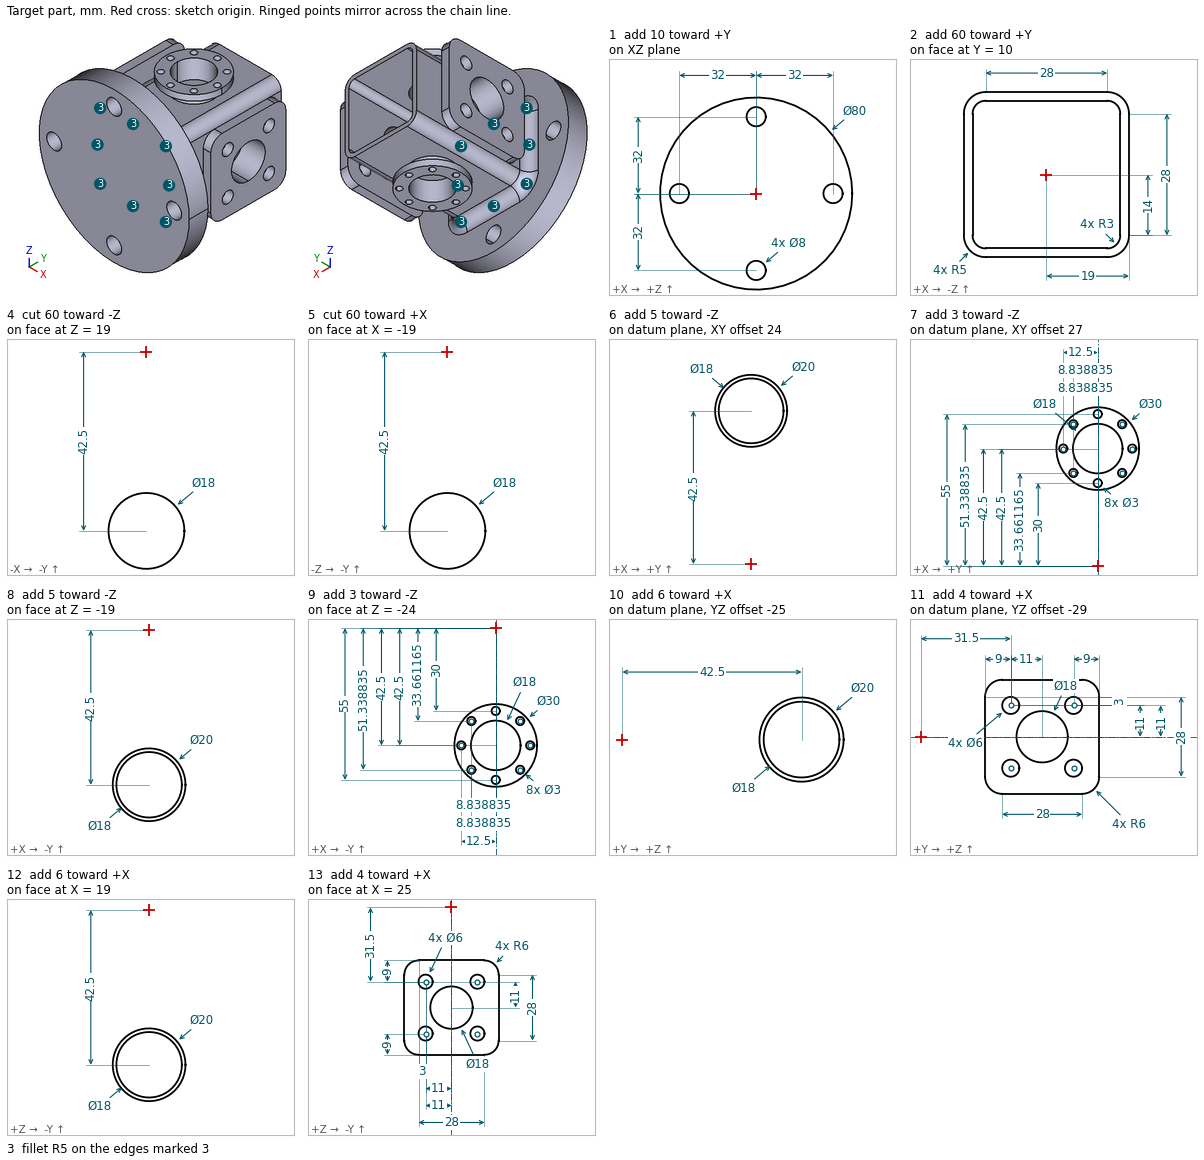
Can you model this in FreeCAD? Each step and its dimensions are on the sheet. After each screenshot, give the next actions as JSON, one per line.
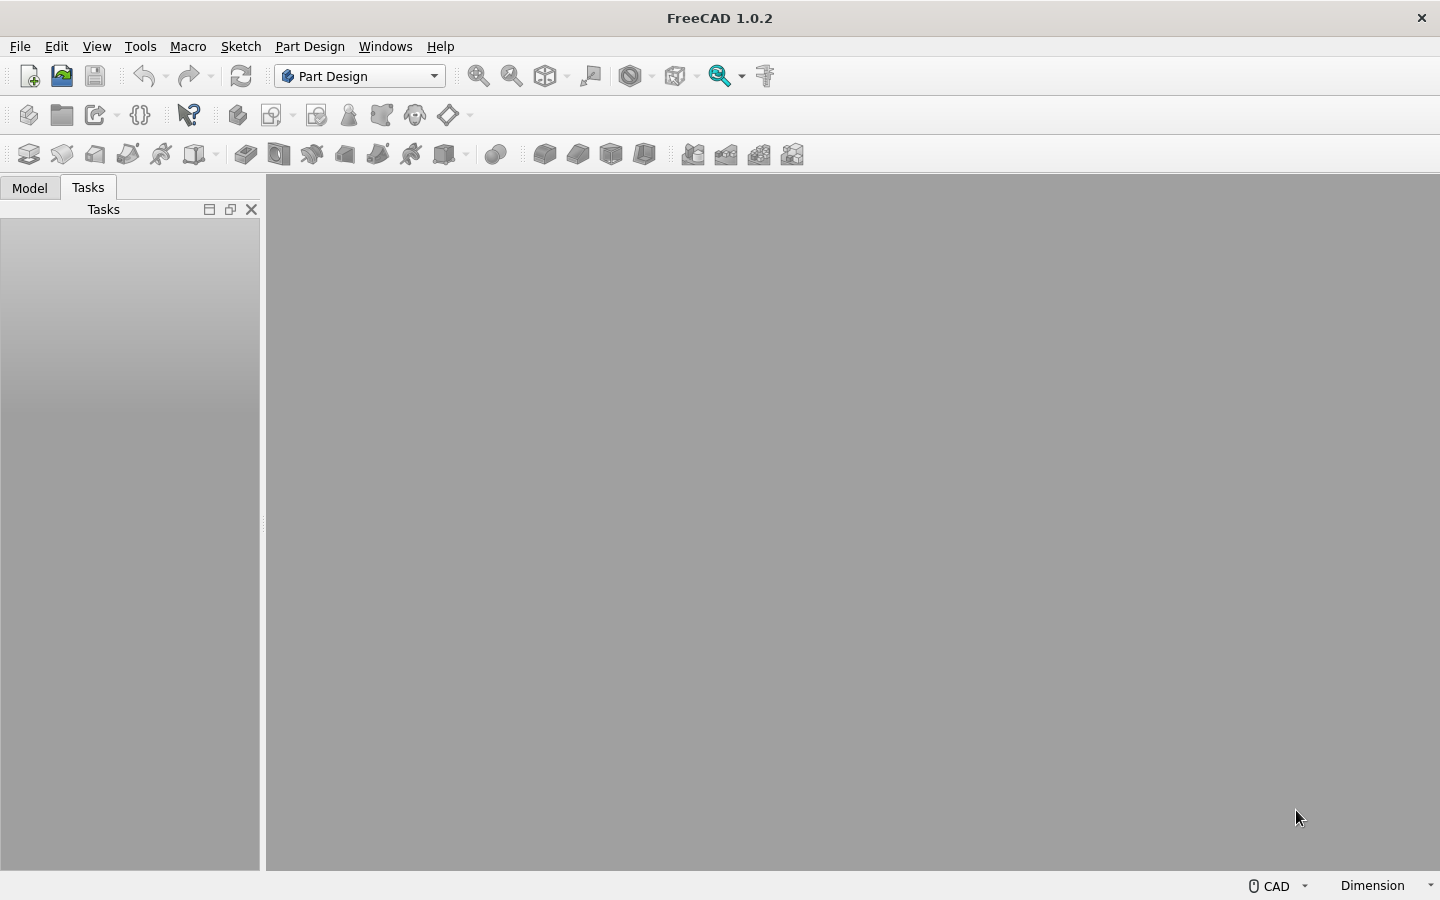
{"action": "key", "text": "ctrl+n"}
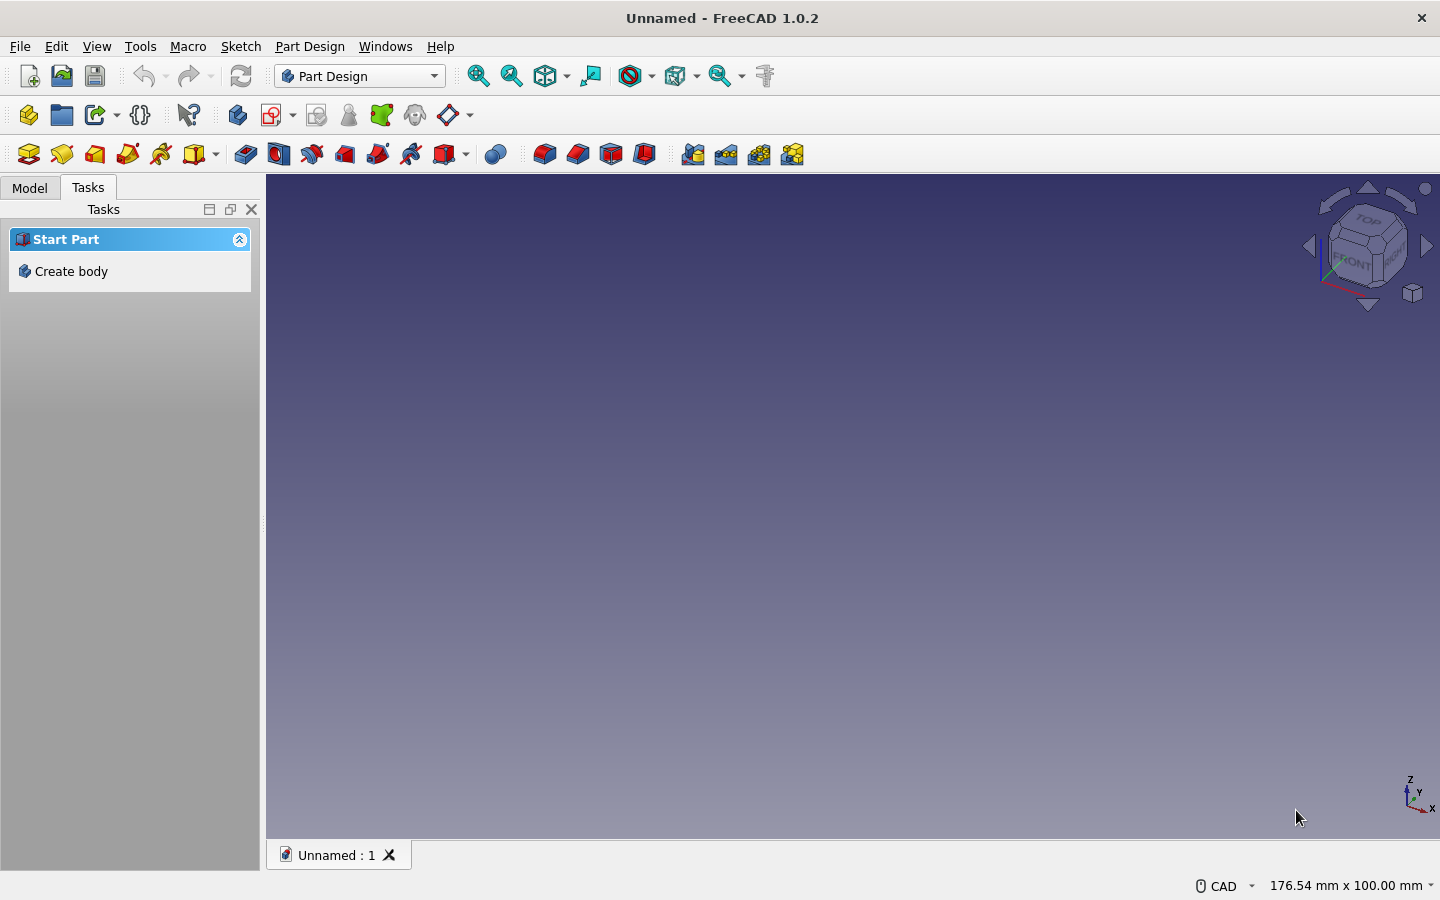
{"action": "left_click", "coordinate": [270, 116]}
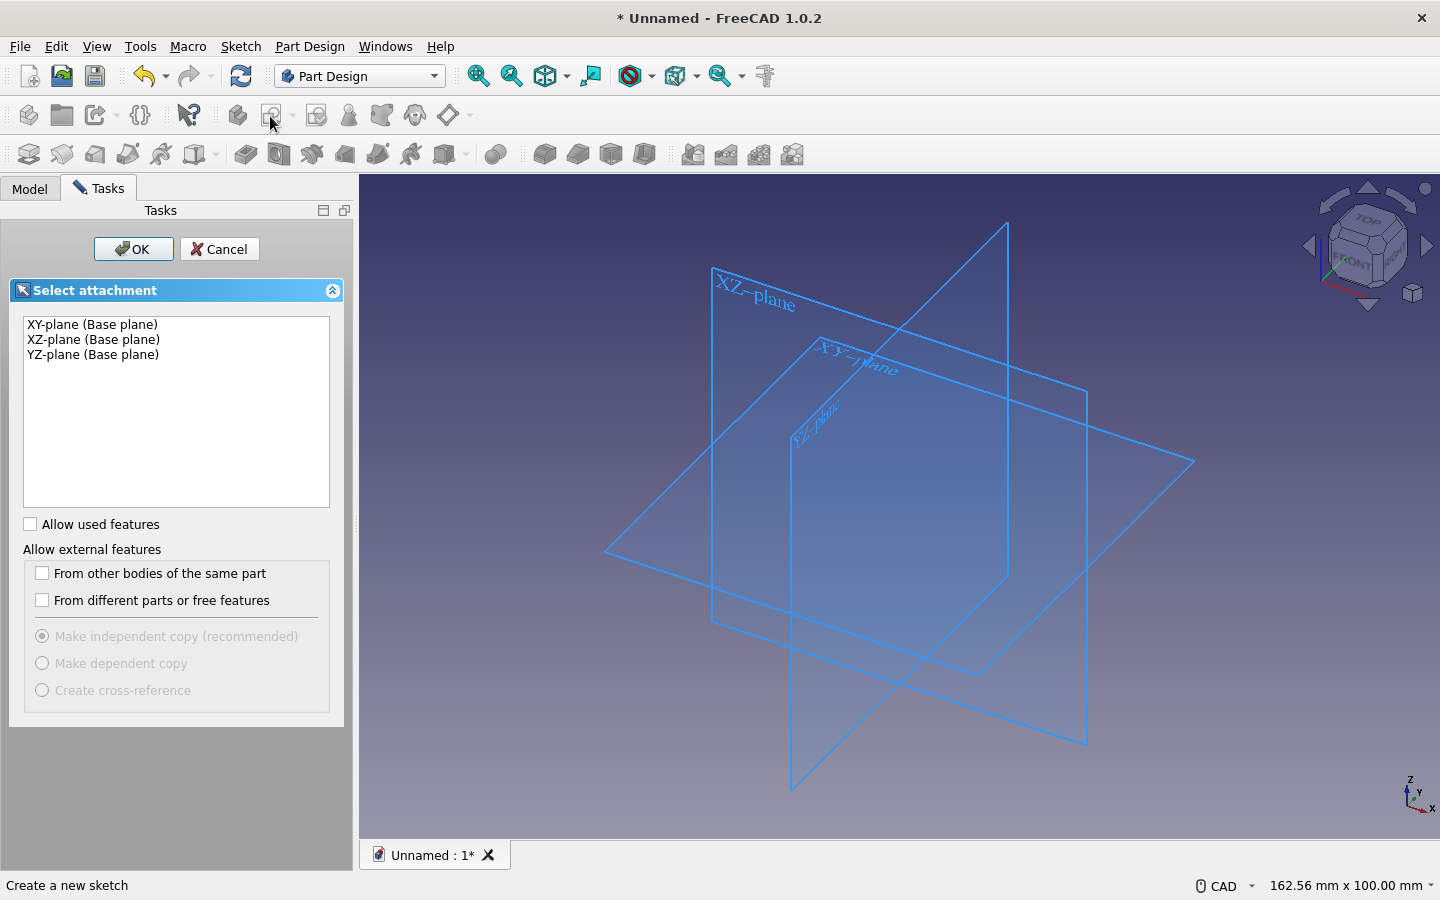
{"action": "left_click", "coordinate": [84, 340]}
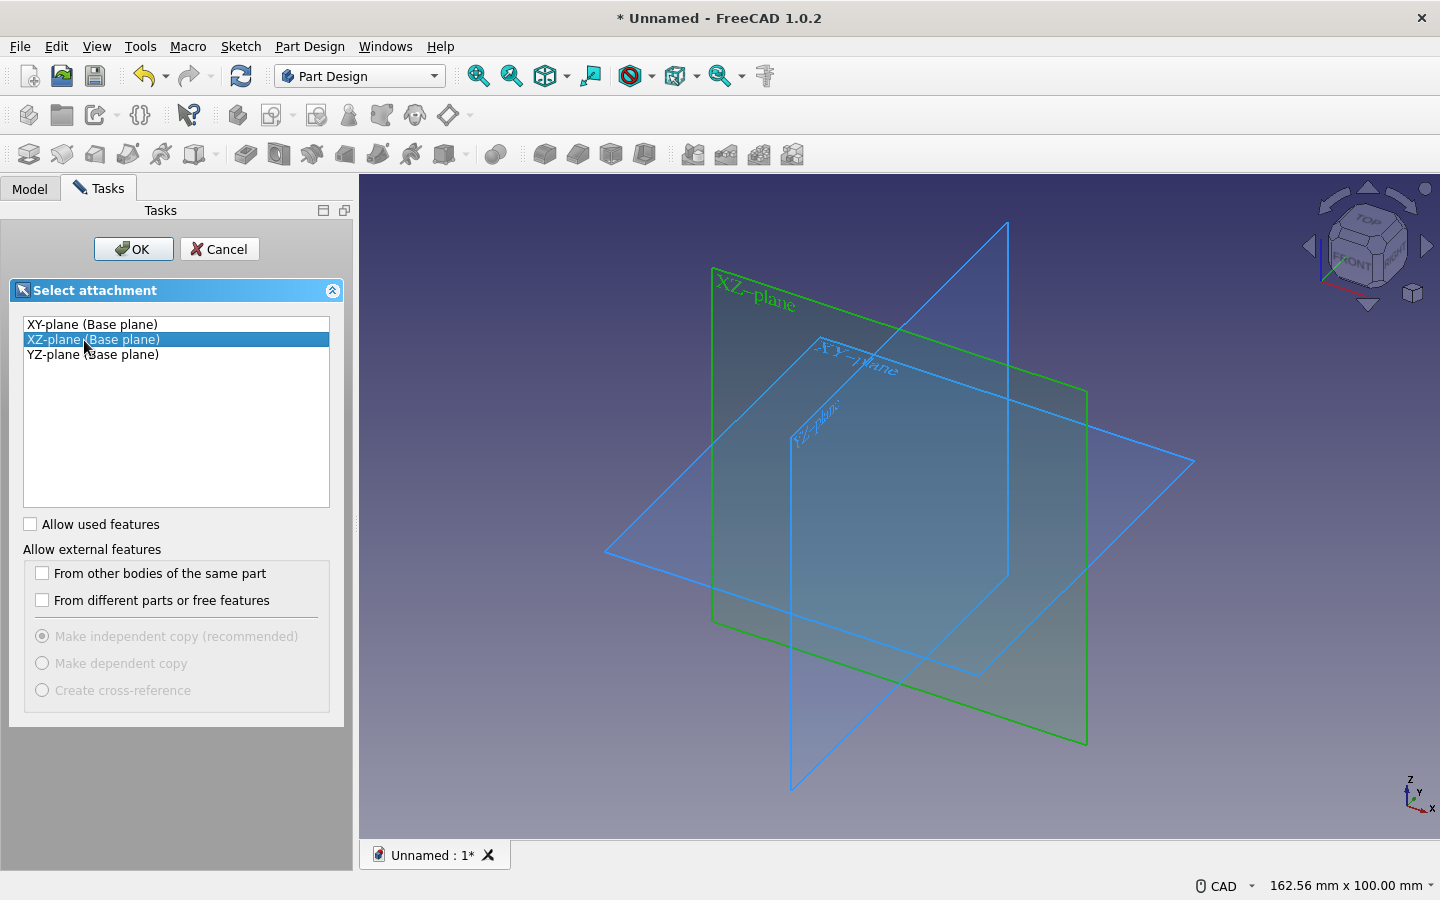
{"action": "left_click", "coordinate": [134, 249]}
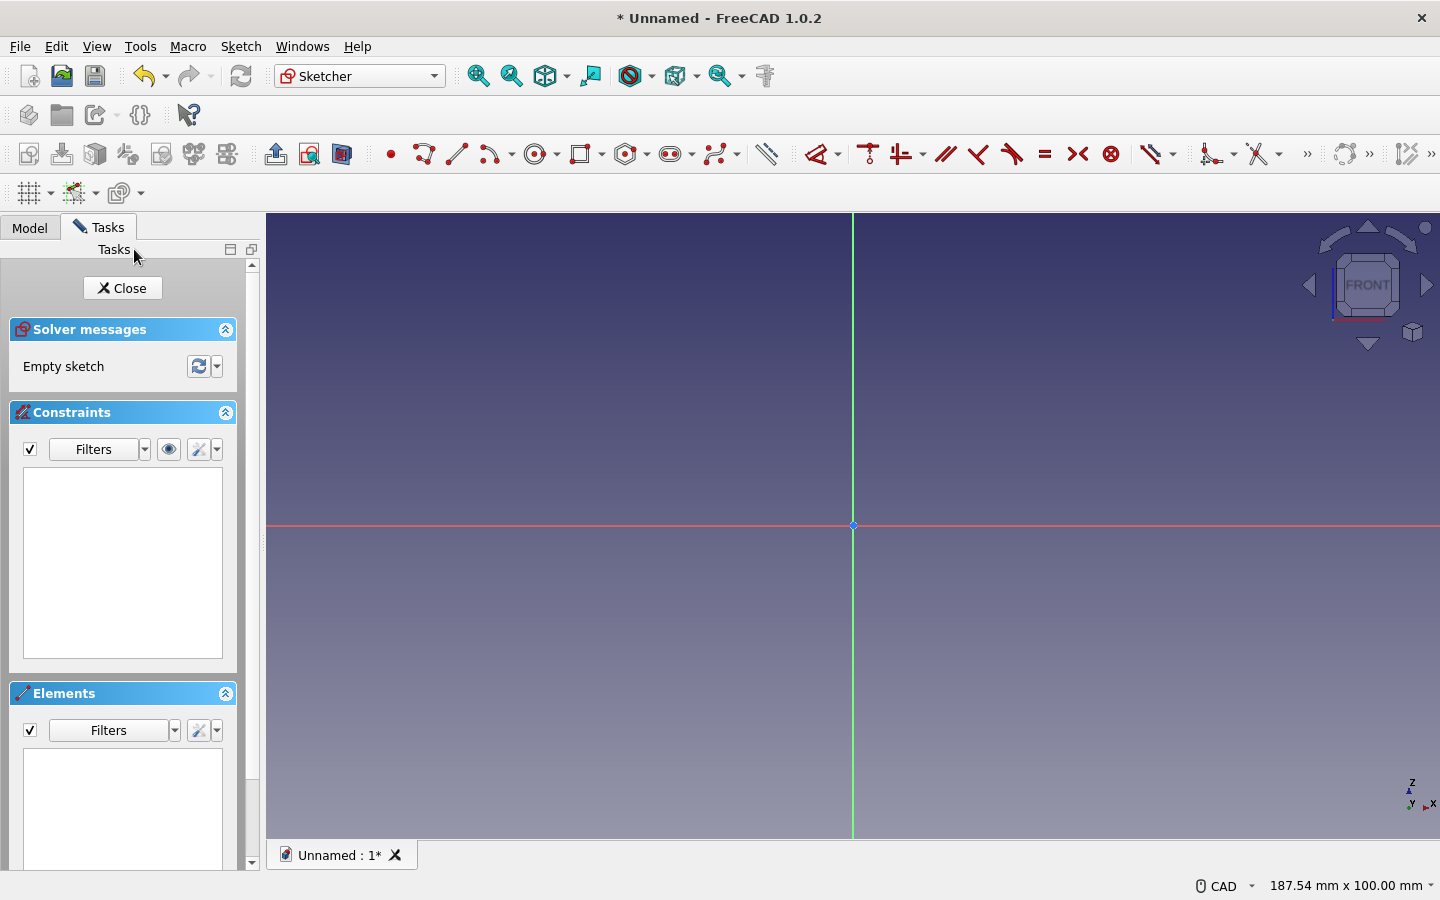
{"action": "left_click", "coordinate": [534, 154]}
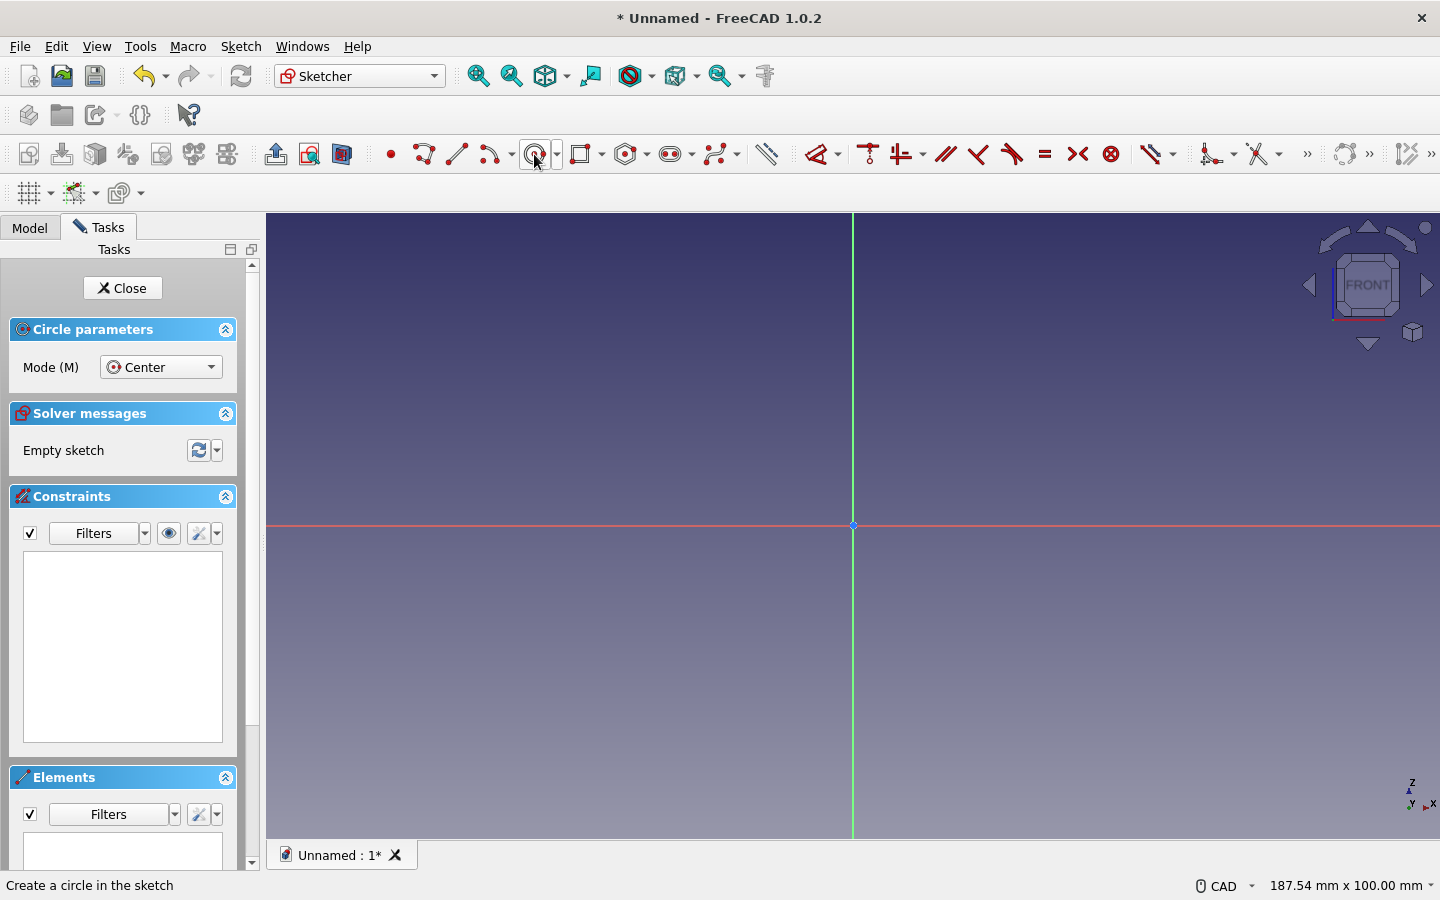
{"action": "left_click", "coordinate": [853, 526]}
{"action": "mouse_move", "coordinate": [1030, 349]}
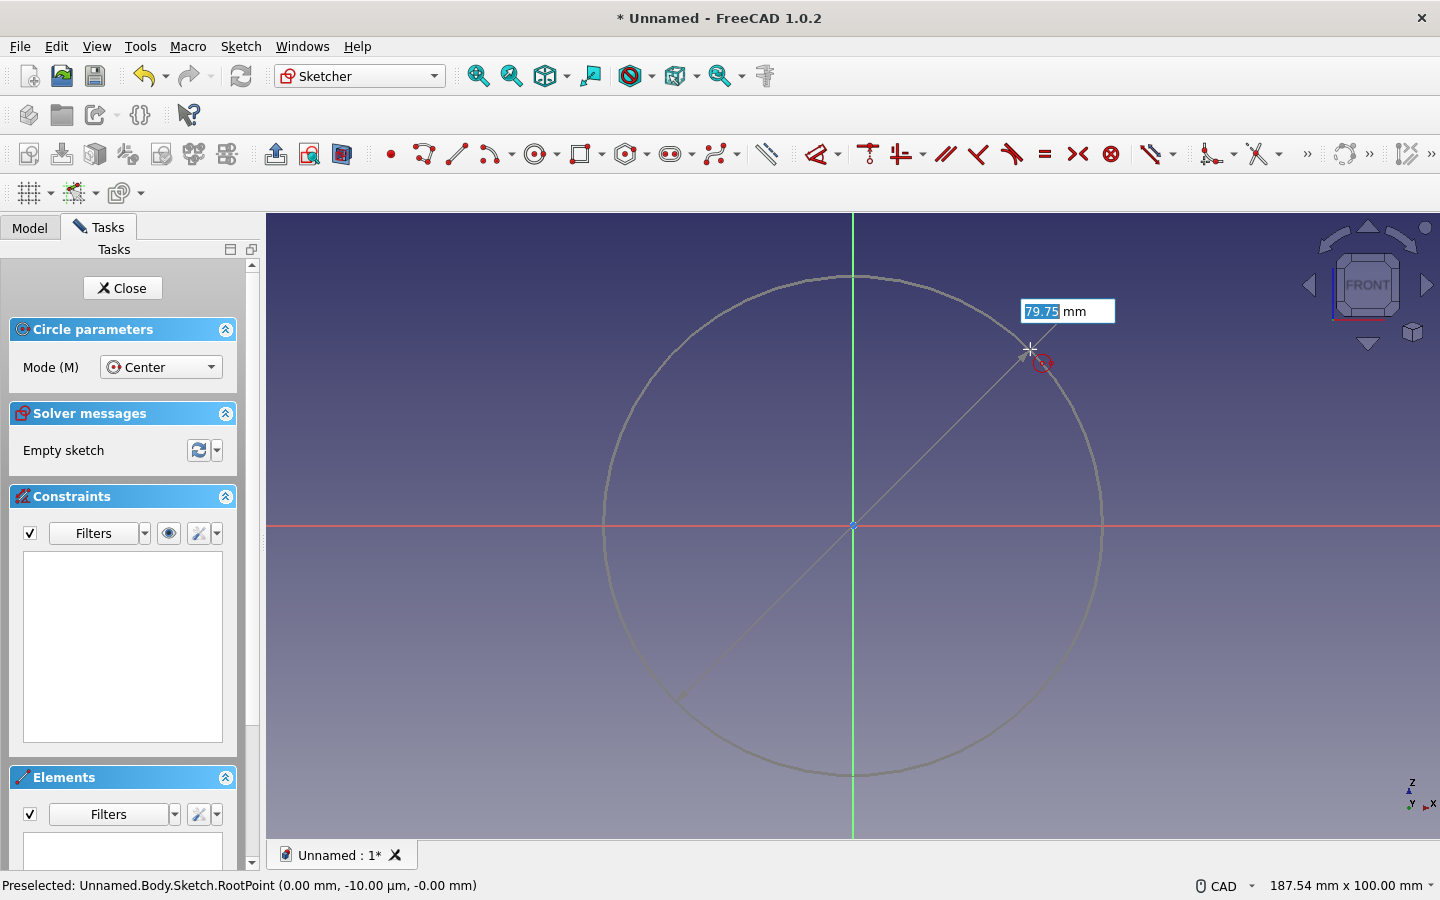
{"action": "type", "text": "80"}
{"action": "key", "text": "Return"}